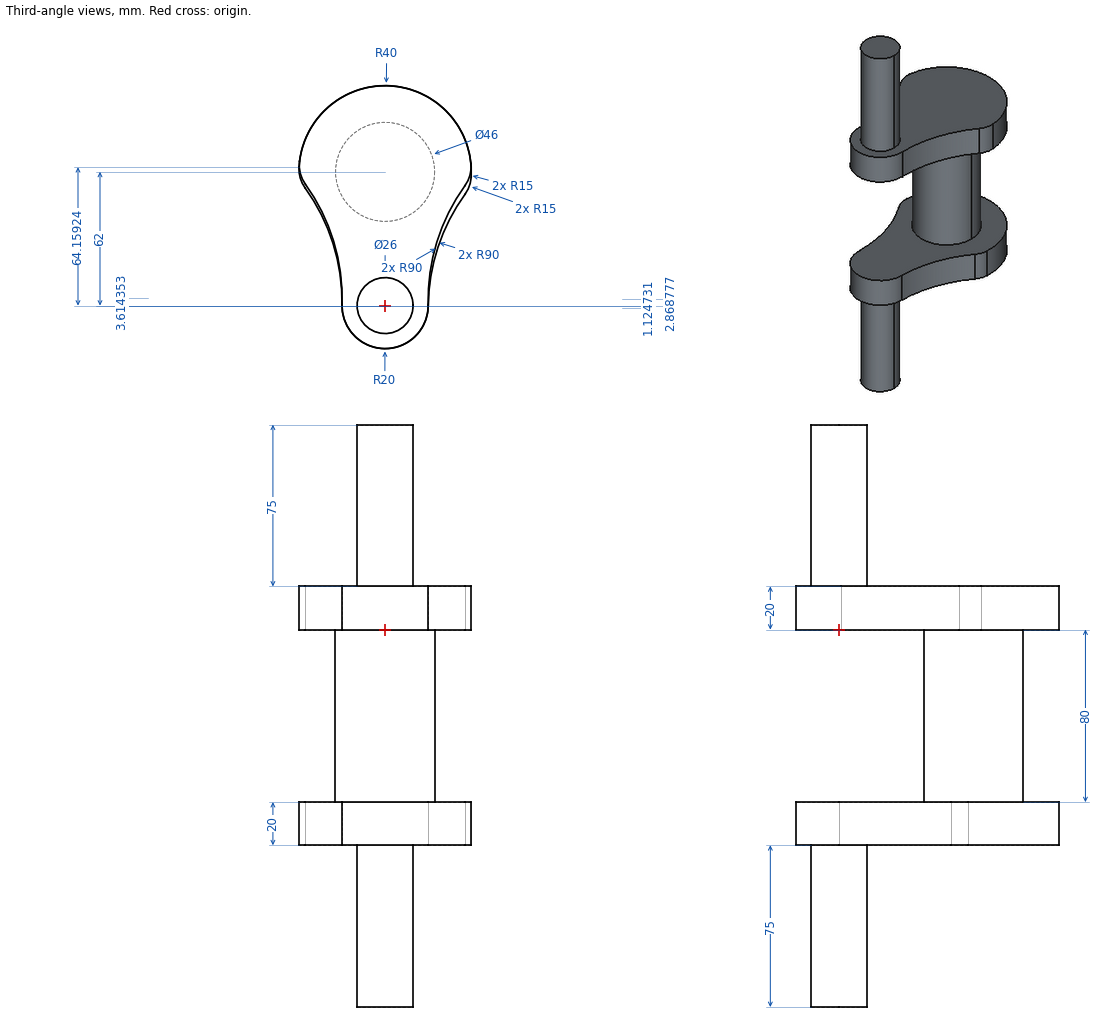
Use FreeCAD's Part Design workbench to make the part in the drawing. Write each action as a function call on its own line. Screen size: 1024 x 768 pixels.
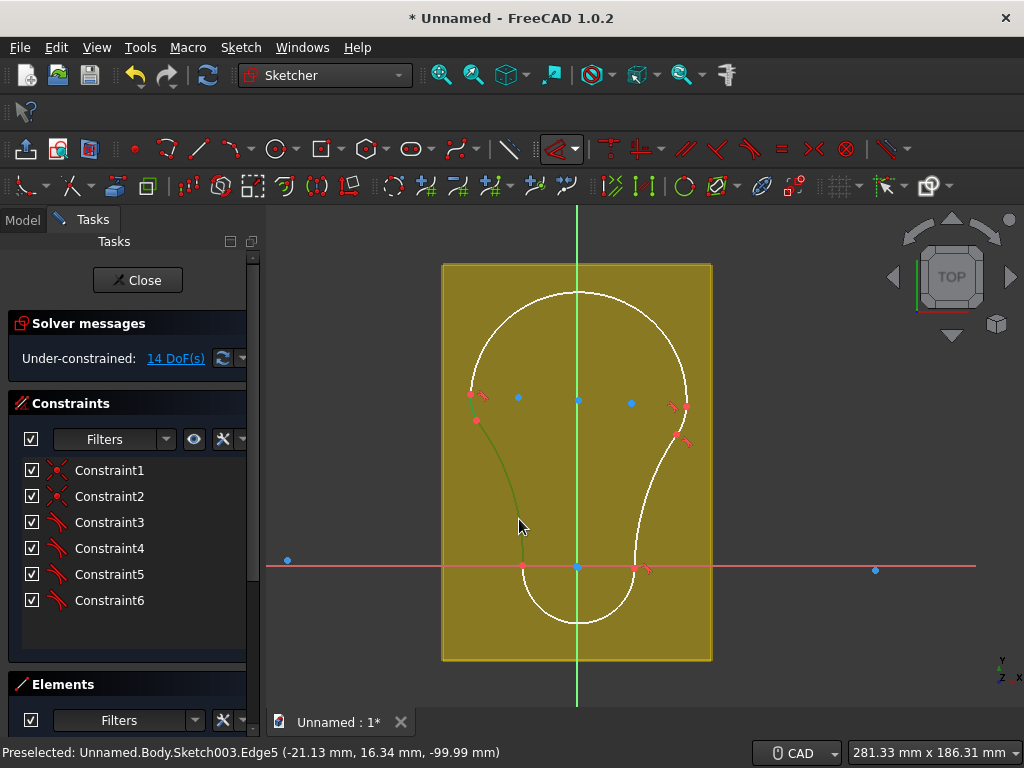
click(750, 150)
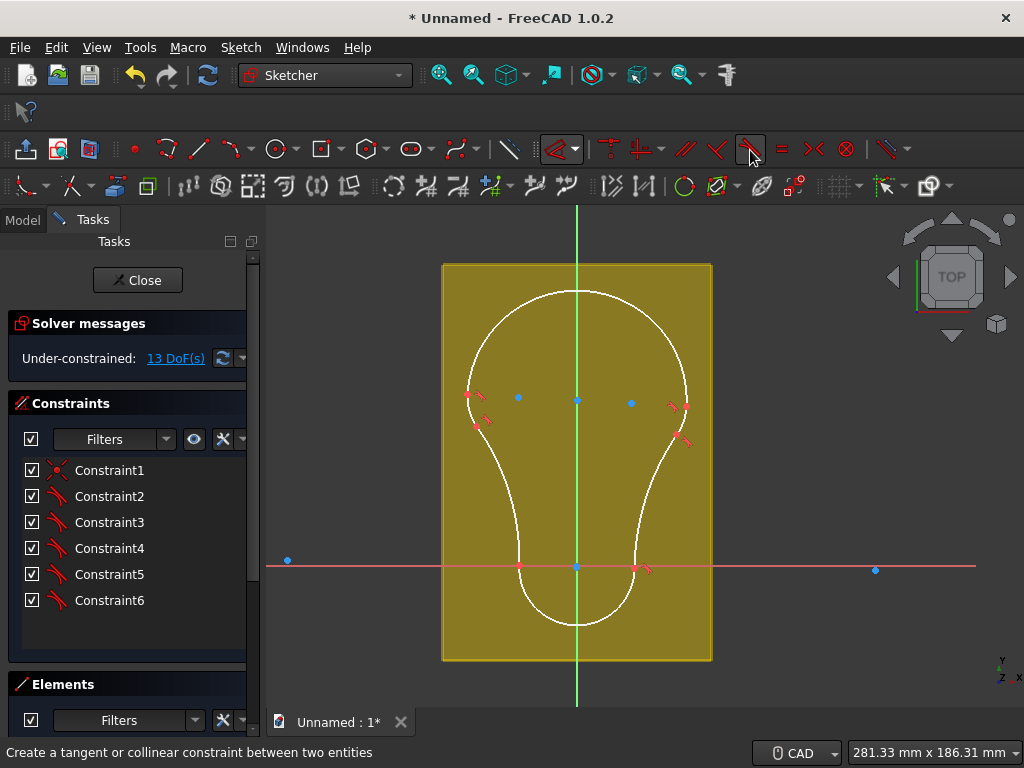
click(516, 522)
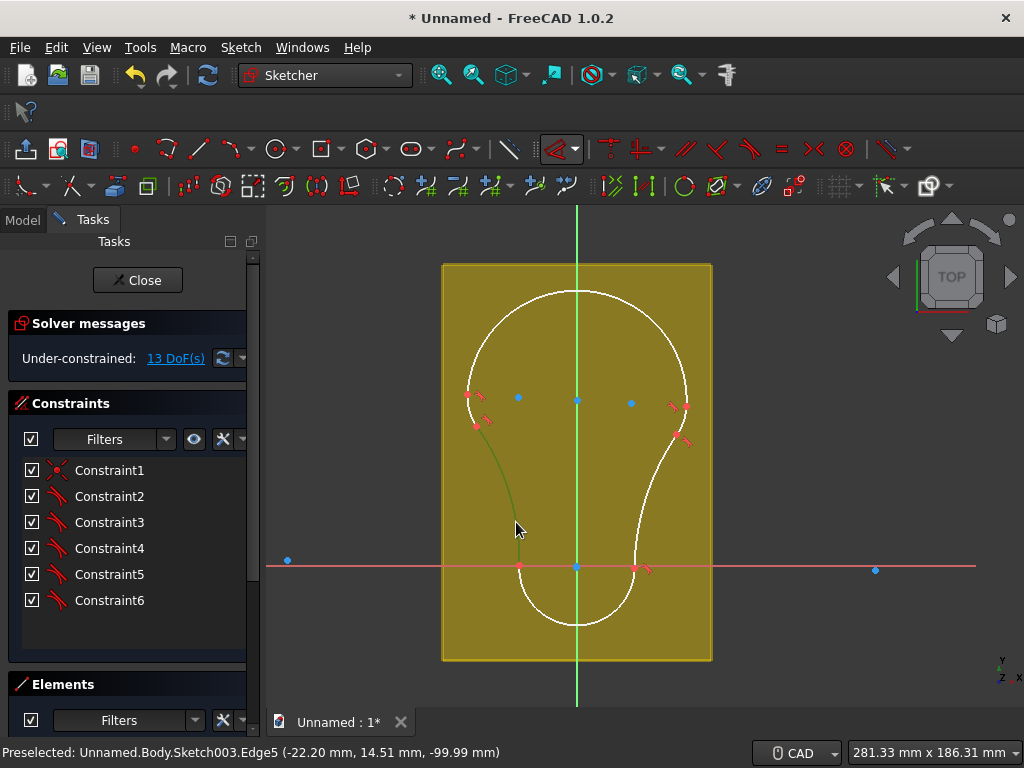
click(542, 613)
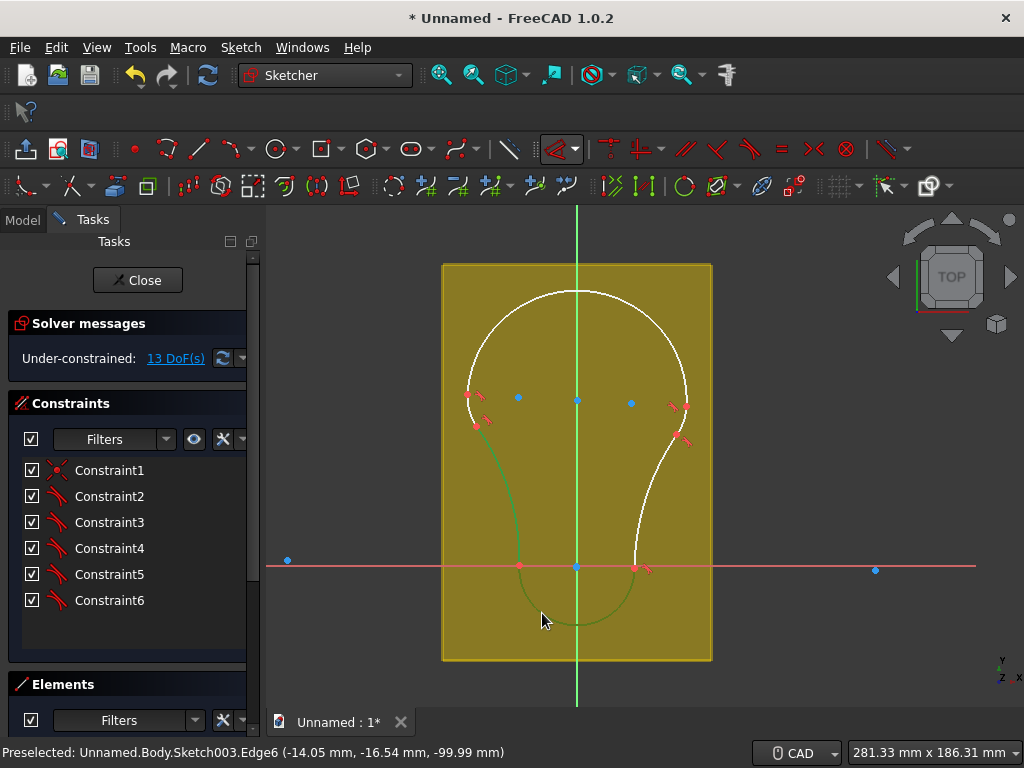
click(750, 150)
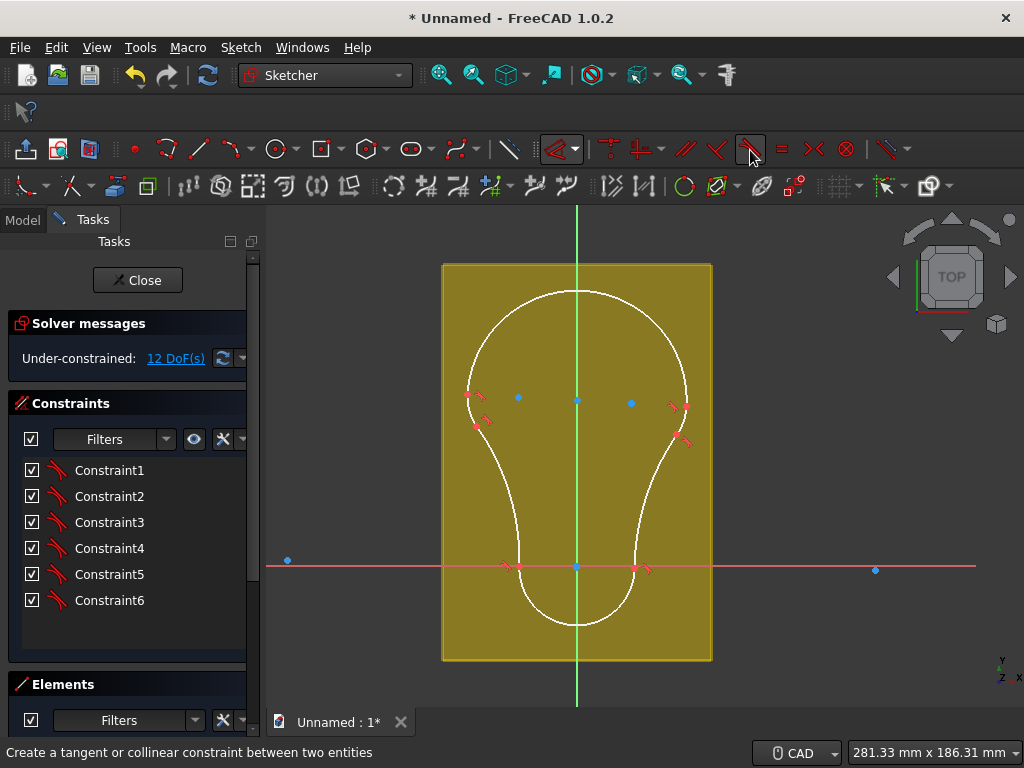
drag(567, 556, 587, 578)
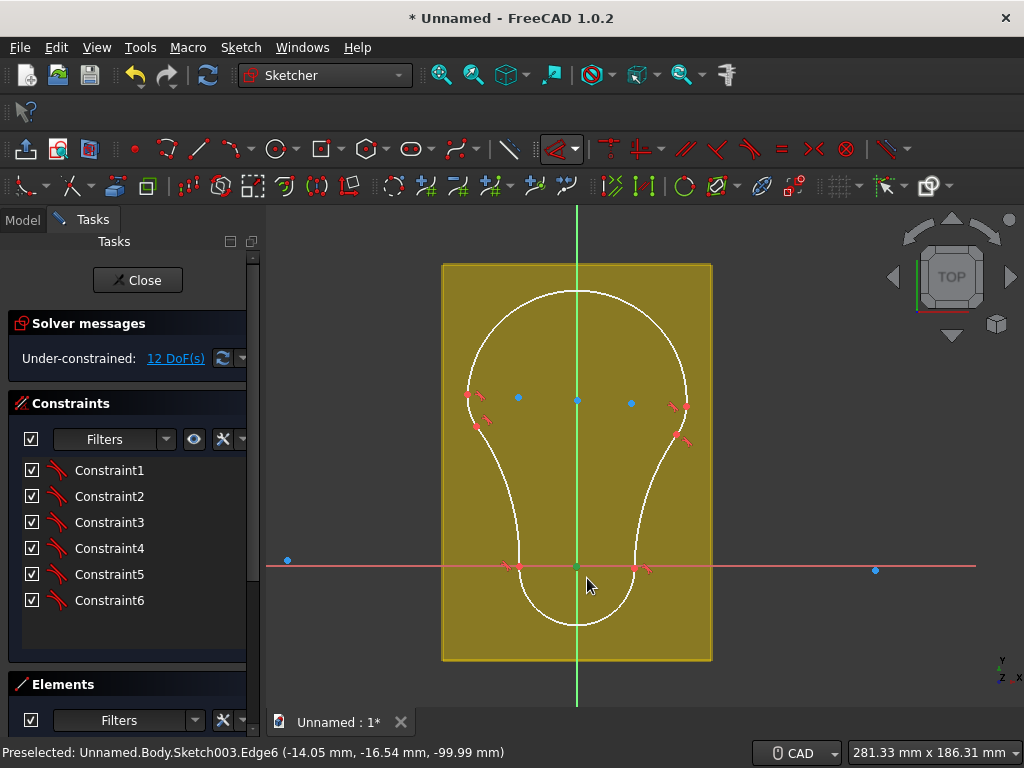
click(610, 150)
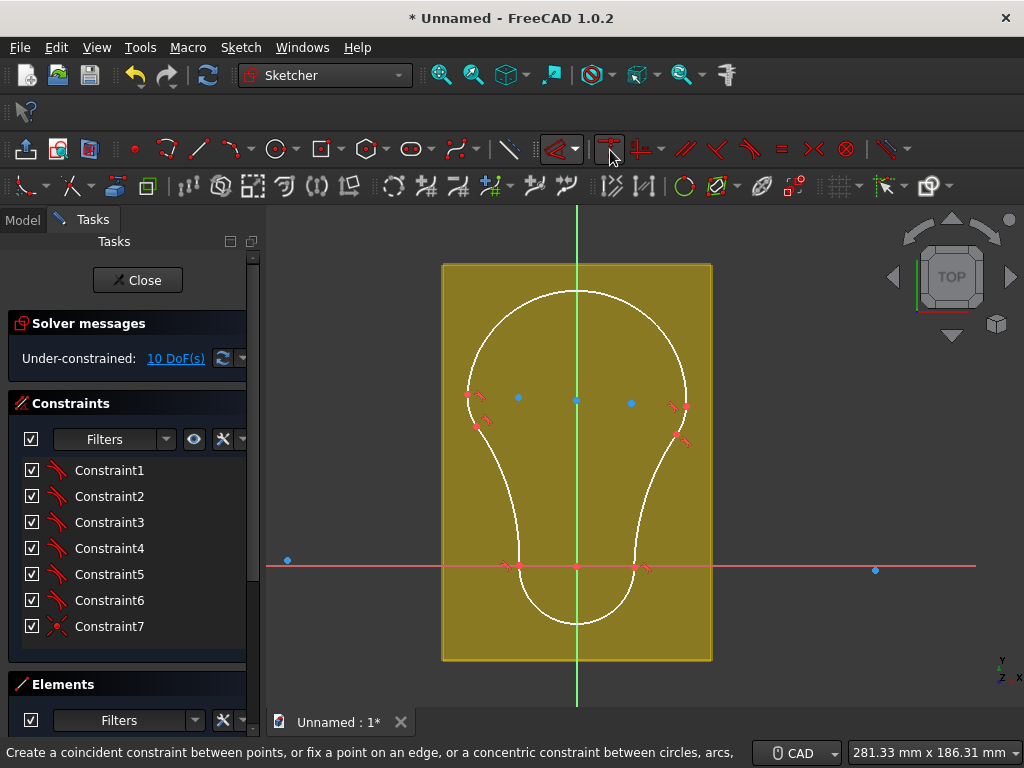
click(683, 421)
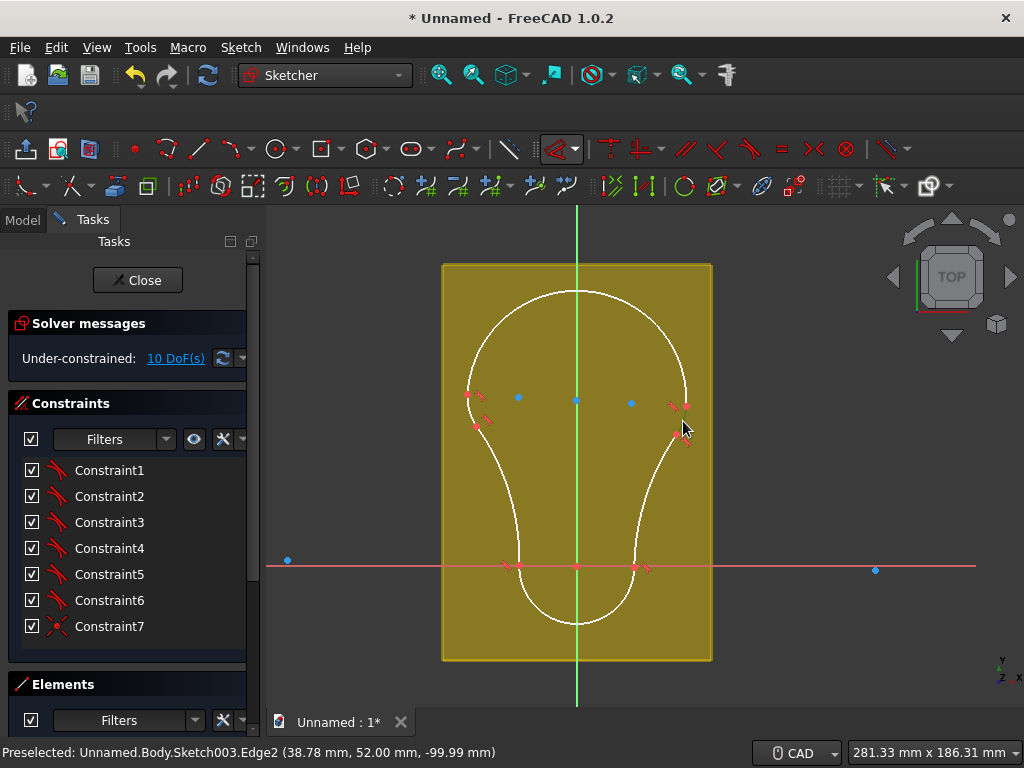
scroll(468, 405, up, 2)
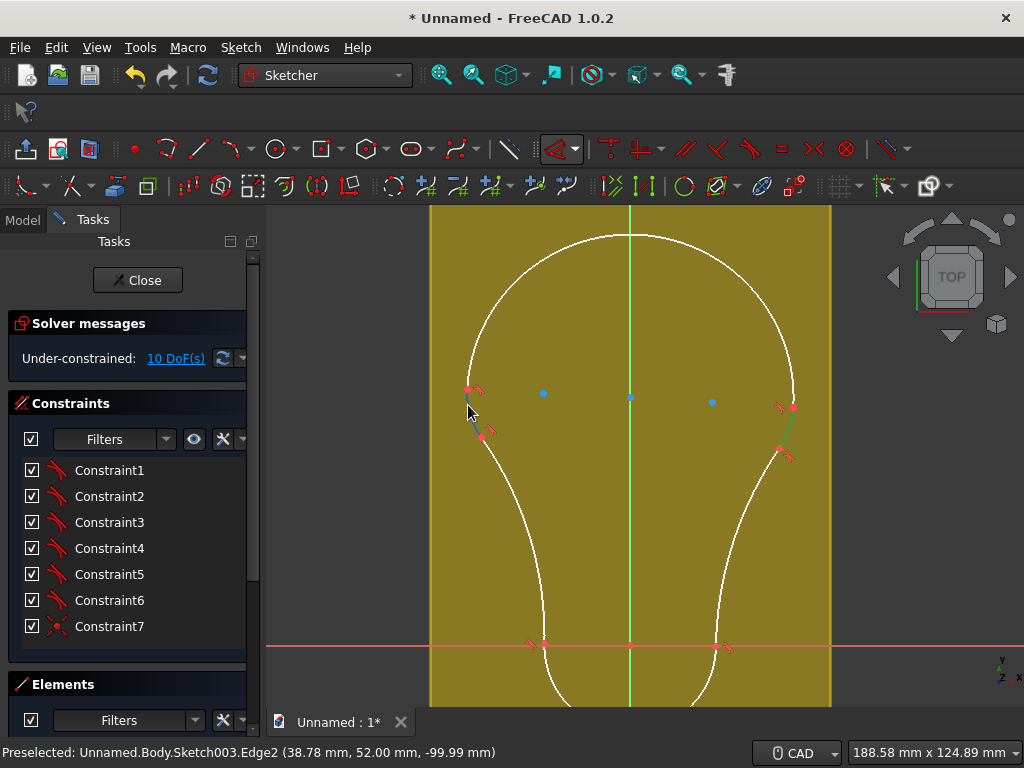
click(468, 404)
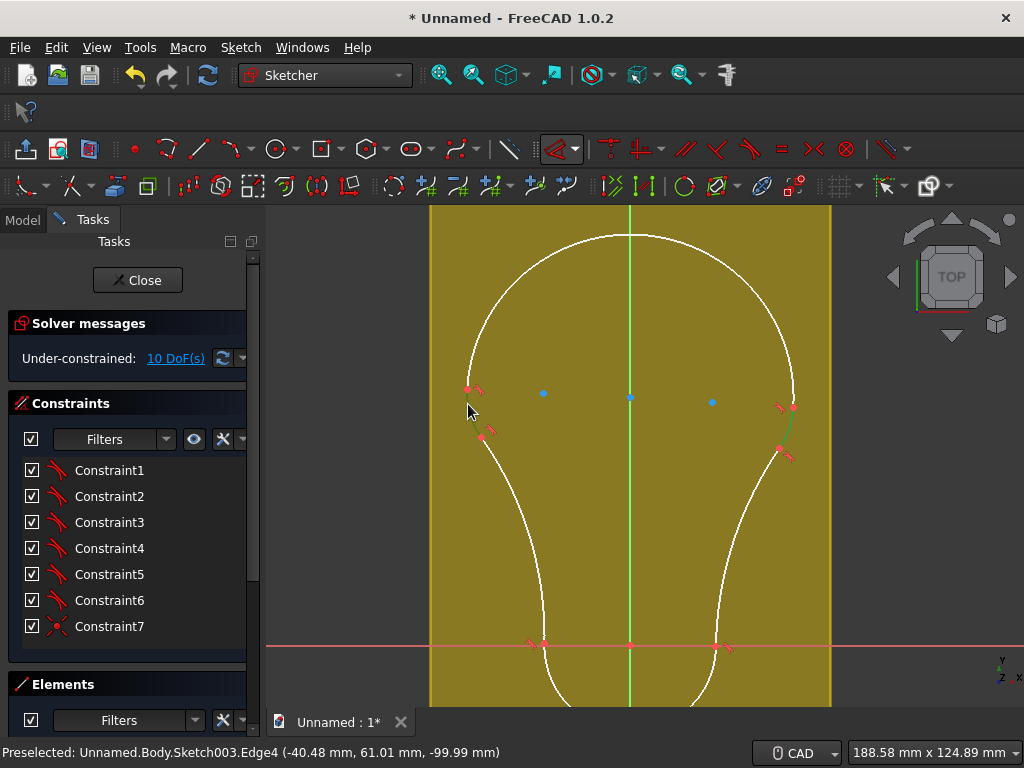
click(782, 150)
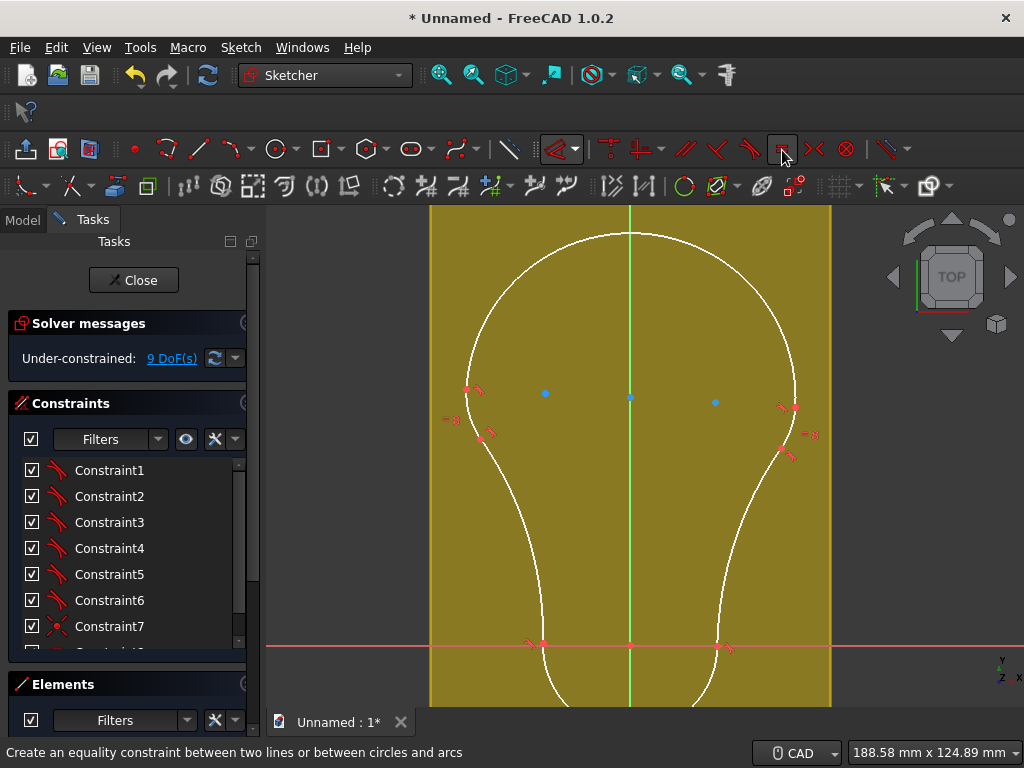
click(750, 503)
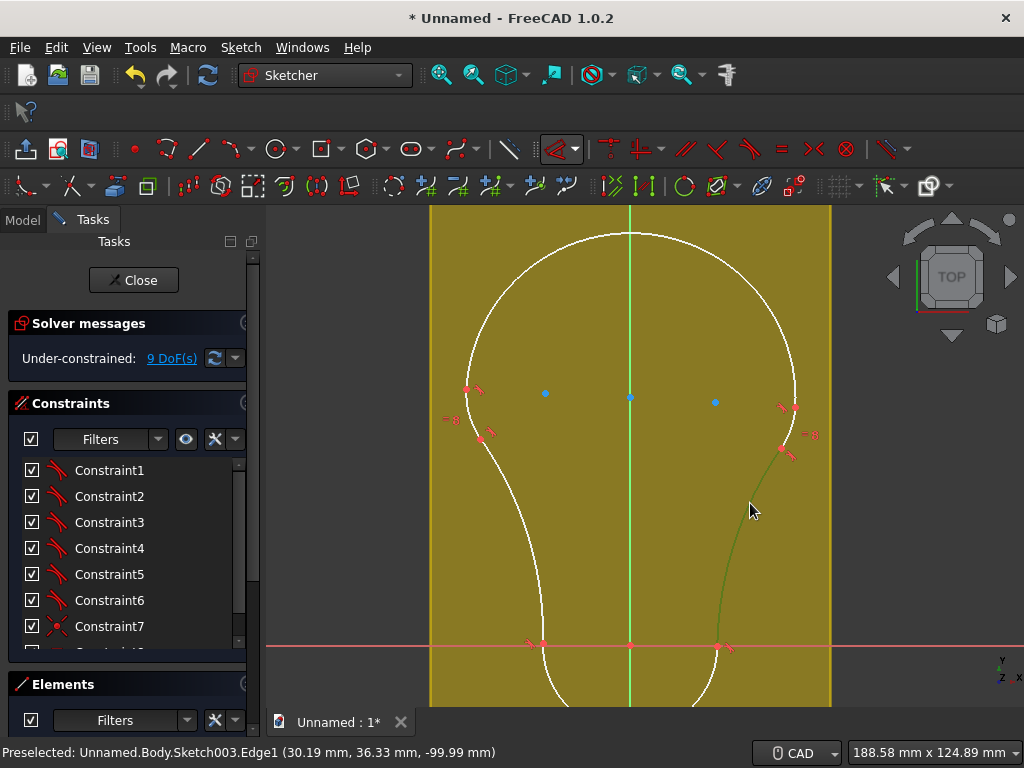
click(538, 579)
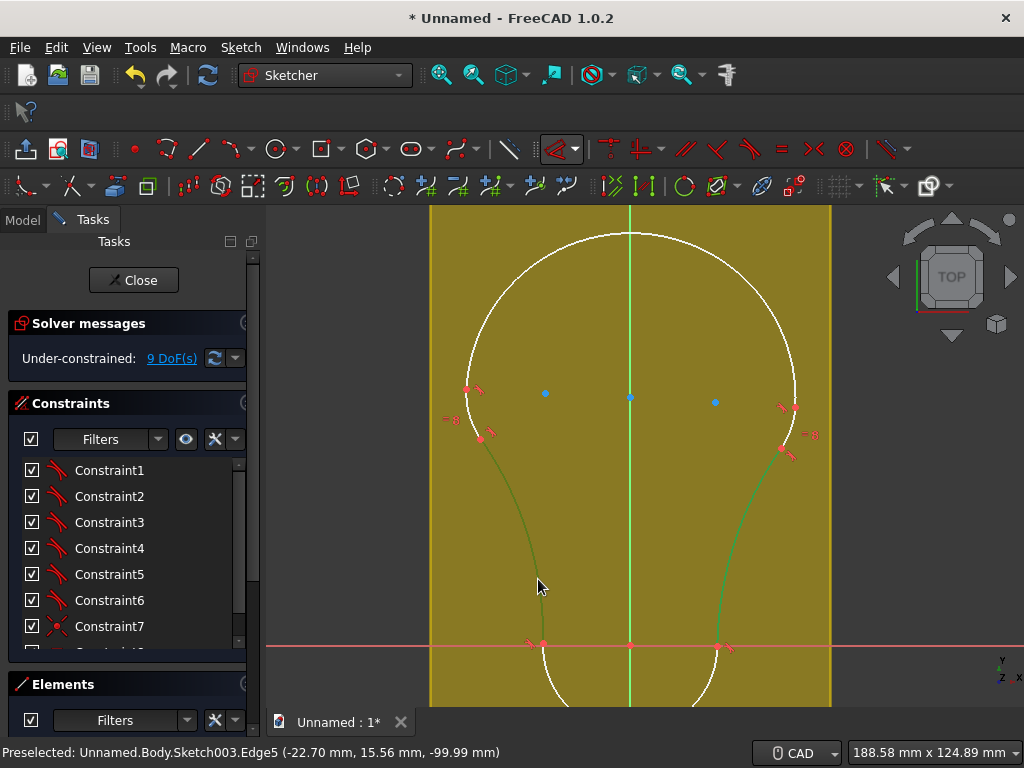
key(e)